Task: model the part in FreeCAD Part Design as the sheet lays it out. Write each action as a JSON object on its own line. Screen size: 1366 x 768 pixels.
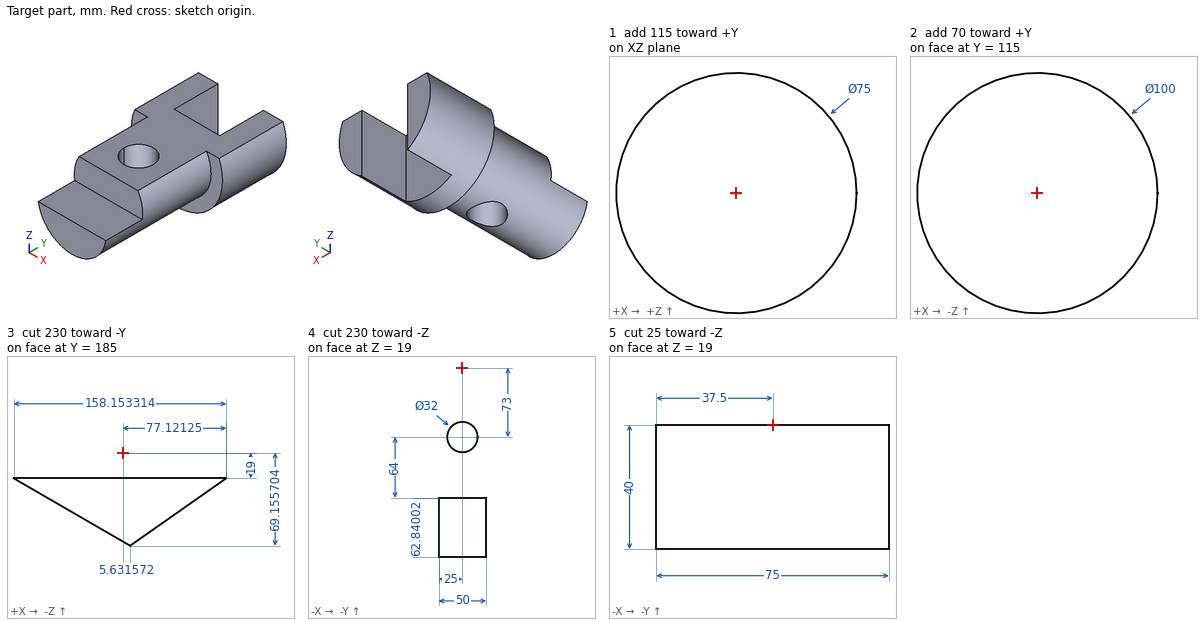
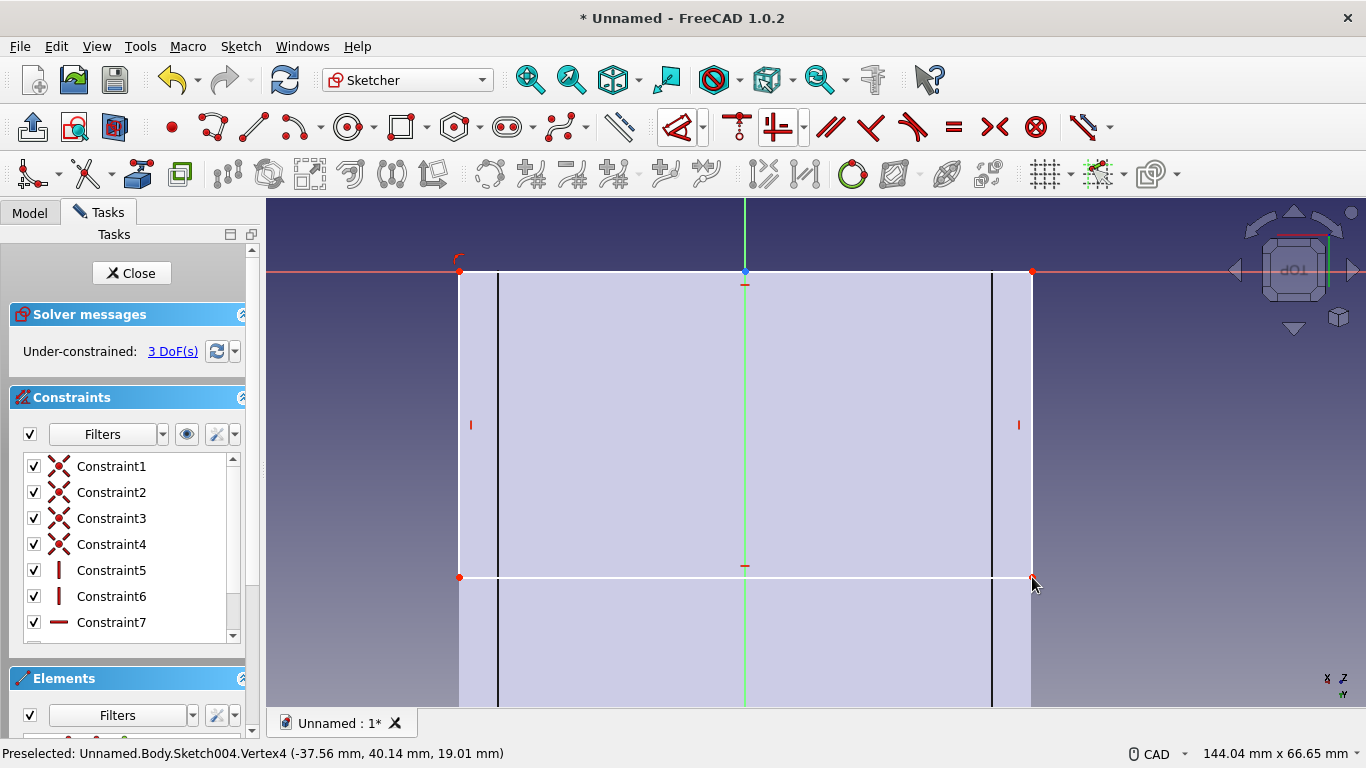
{"action": "left_click", "coordinate": [459, 363]}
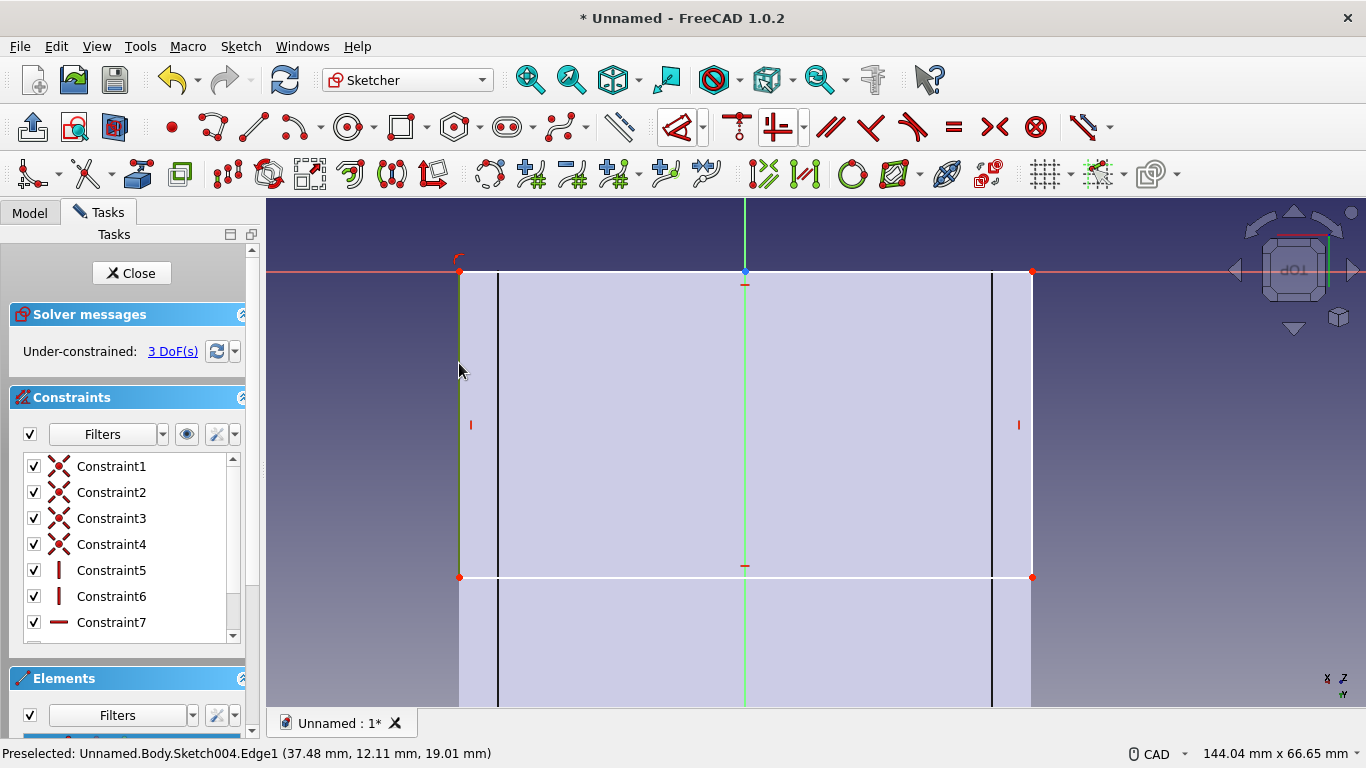
{"action": "left_click", "coordinate": [702, 128]}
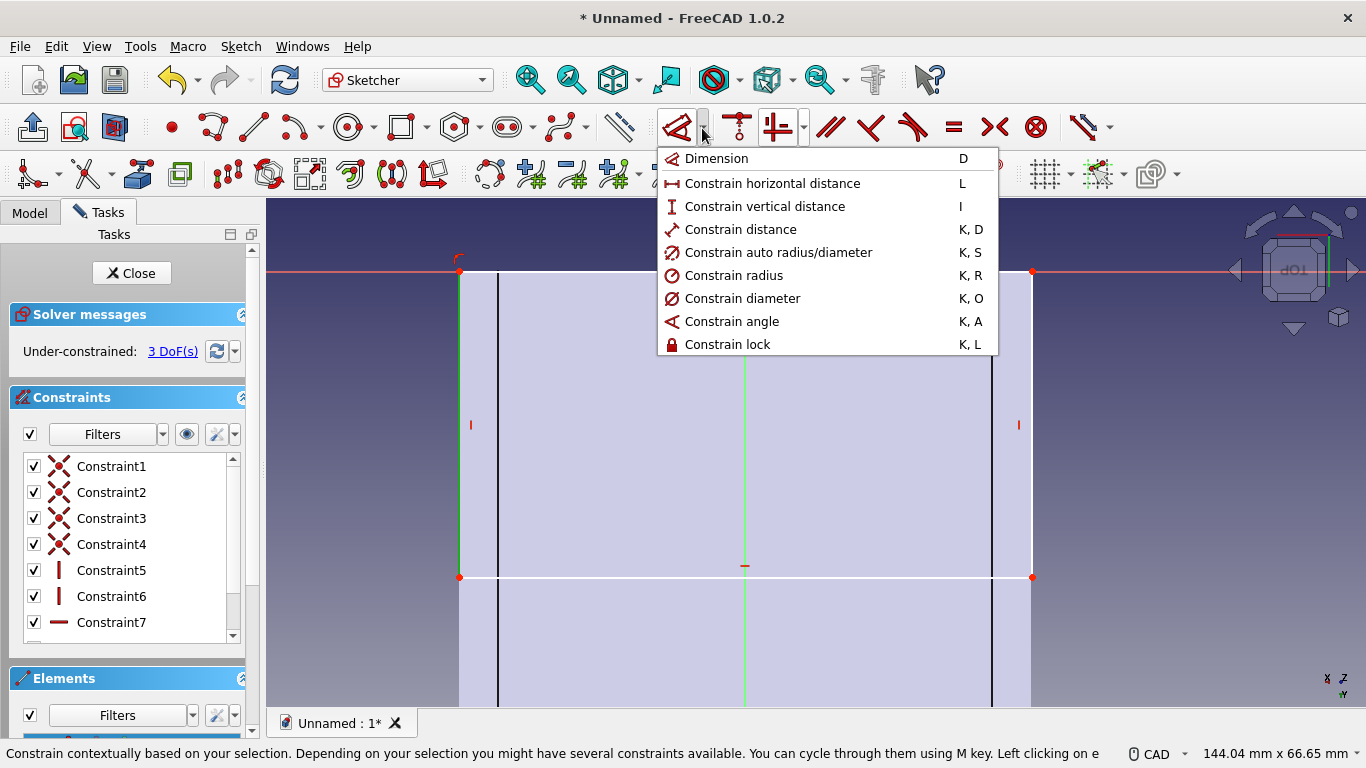
{"action": "left_click", "coordinate": [828, 206]}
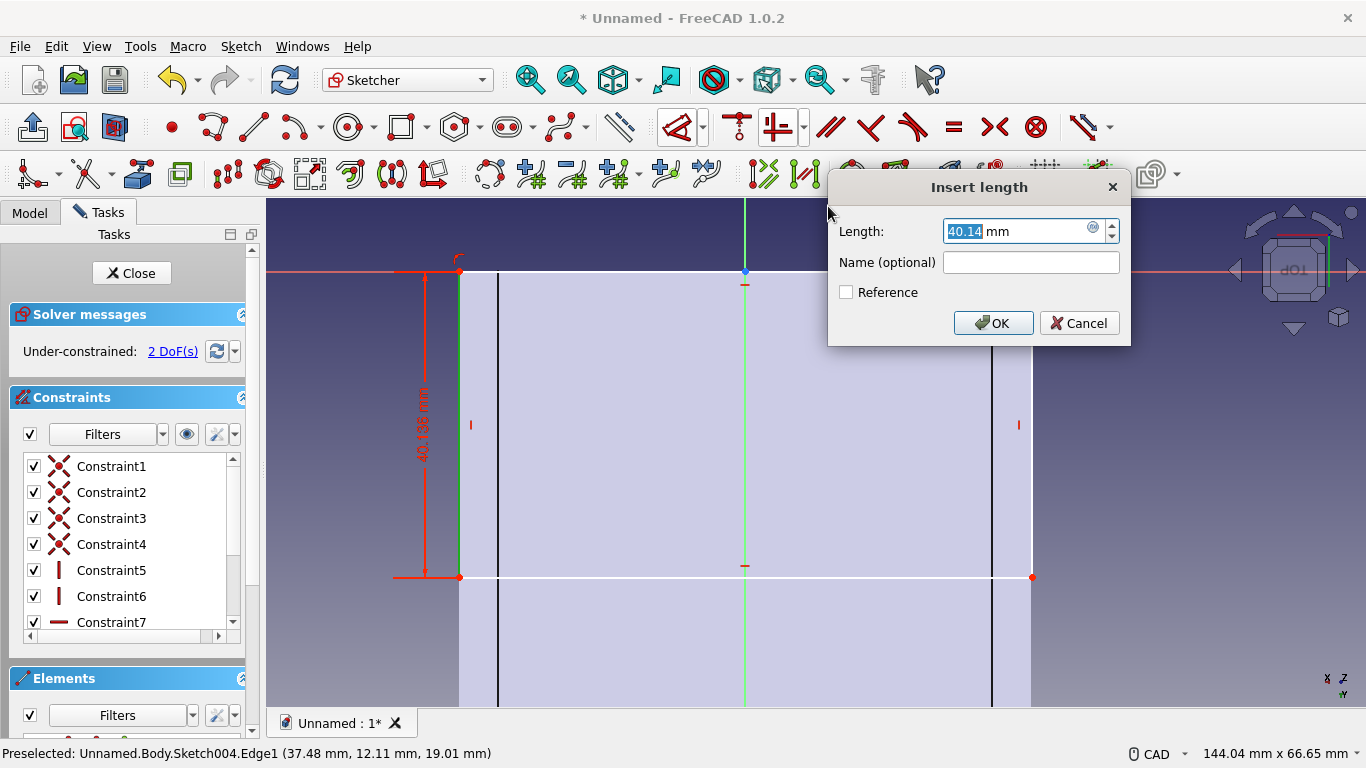
{"action": "type", "text": "40"}
{"action": "key", "text": "Return"}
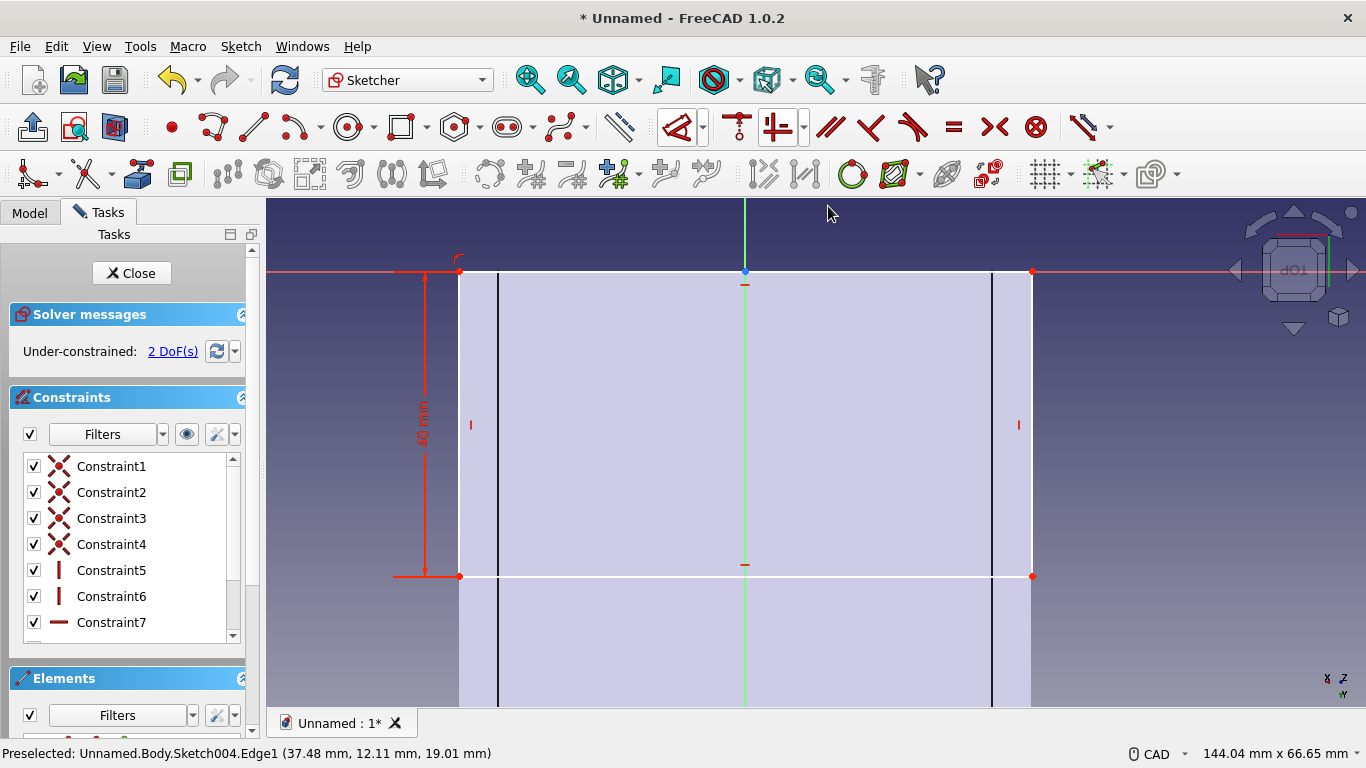
{"action": "left_click", "coordinate": [631, 577]}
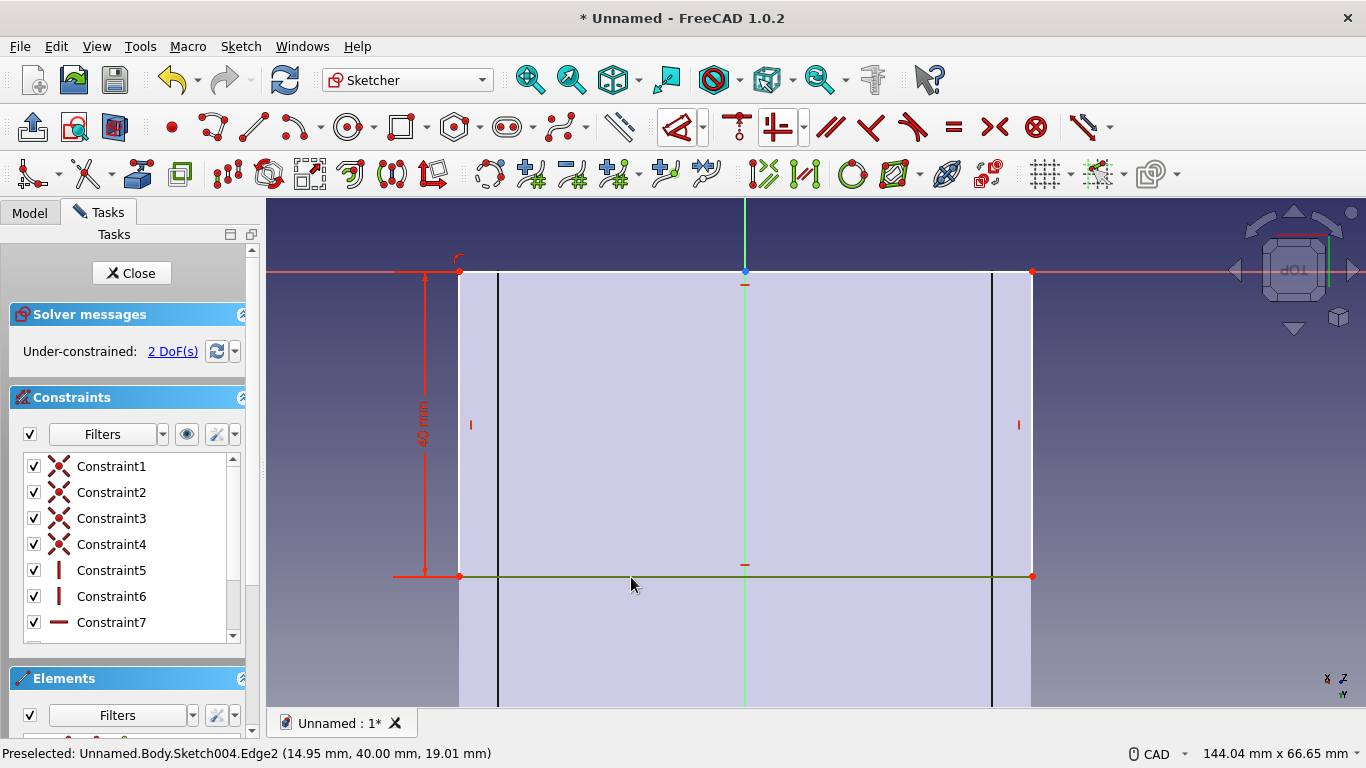
{"action": "left_click", "coordinate": [702, 128]}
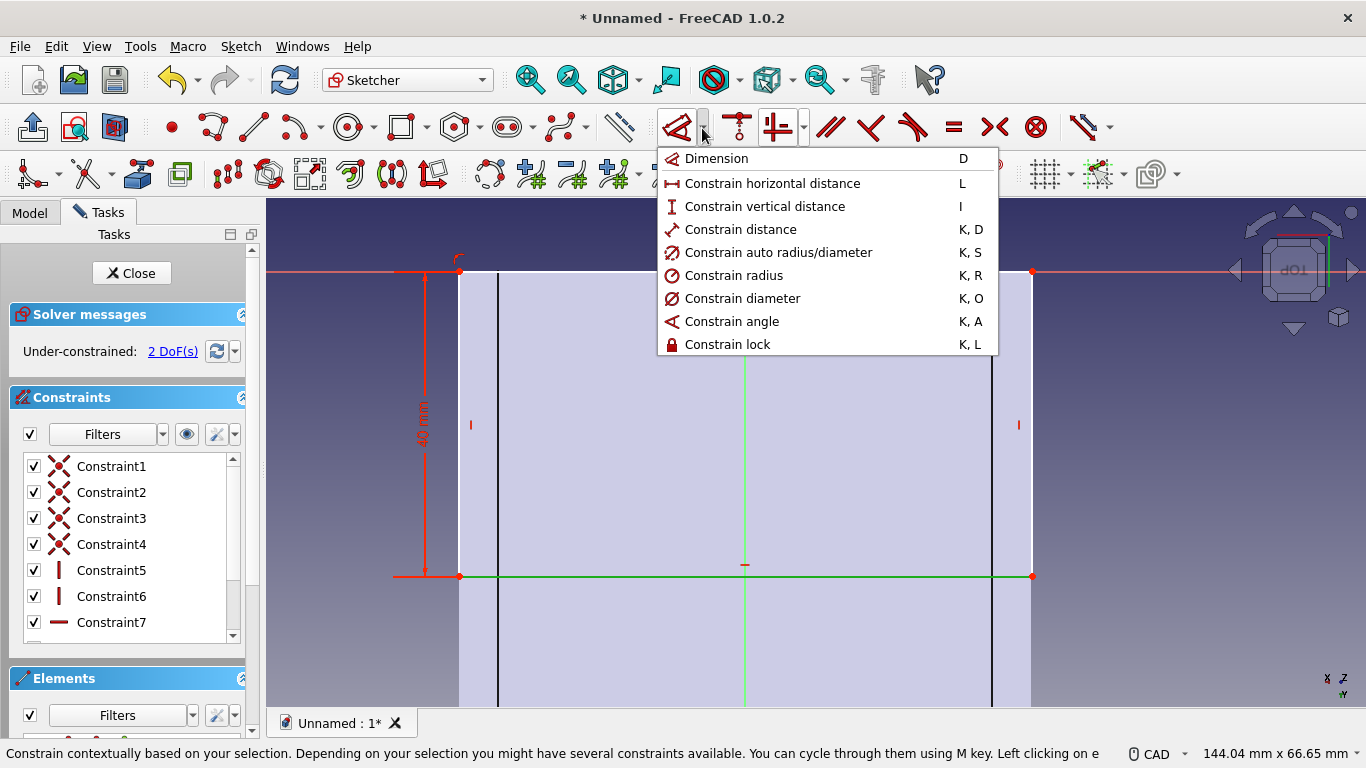
{"action": "left_click", "coordinate": [828, 184]}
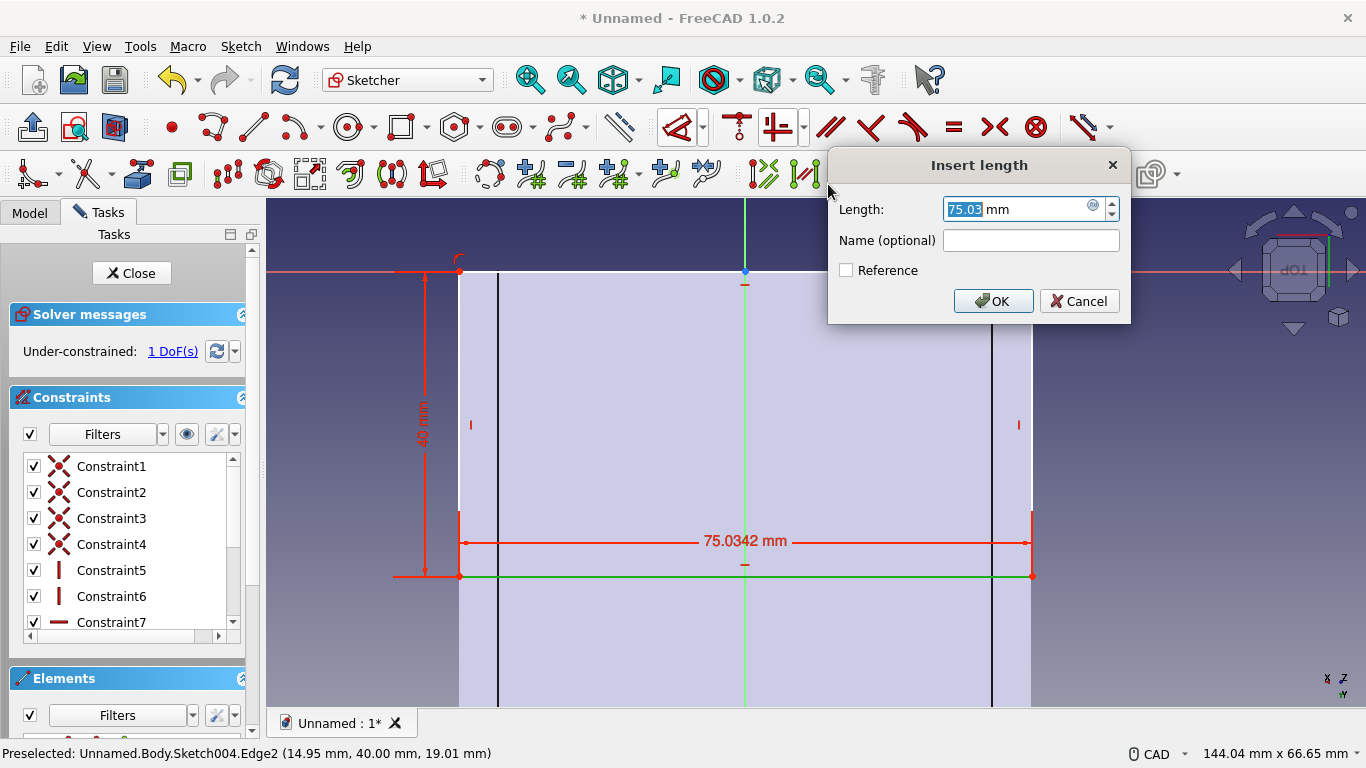
{"action": "type", "text": "75"}
{"action": "key", "text": "Return"}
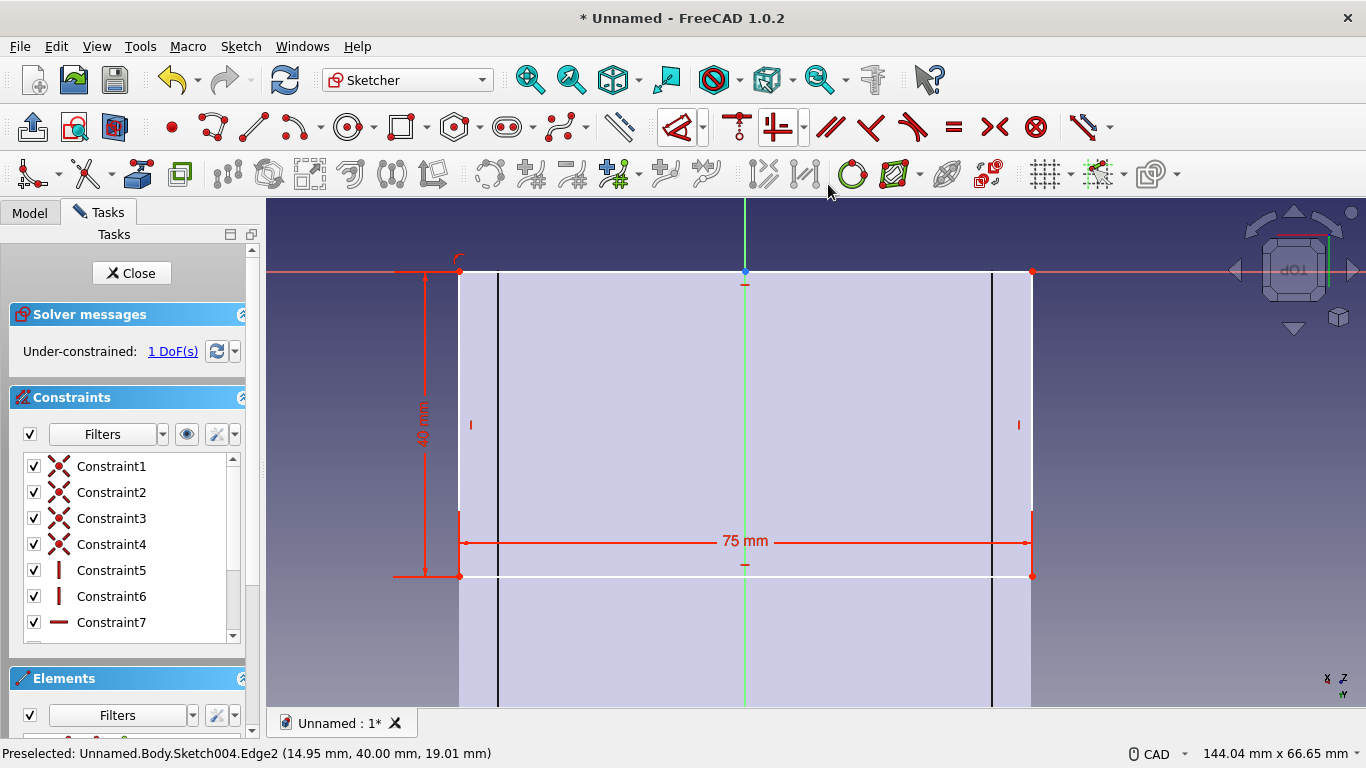
{"action": "left_click", "coordinate": [459, 272]}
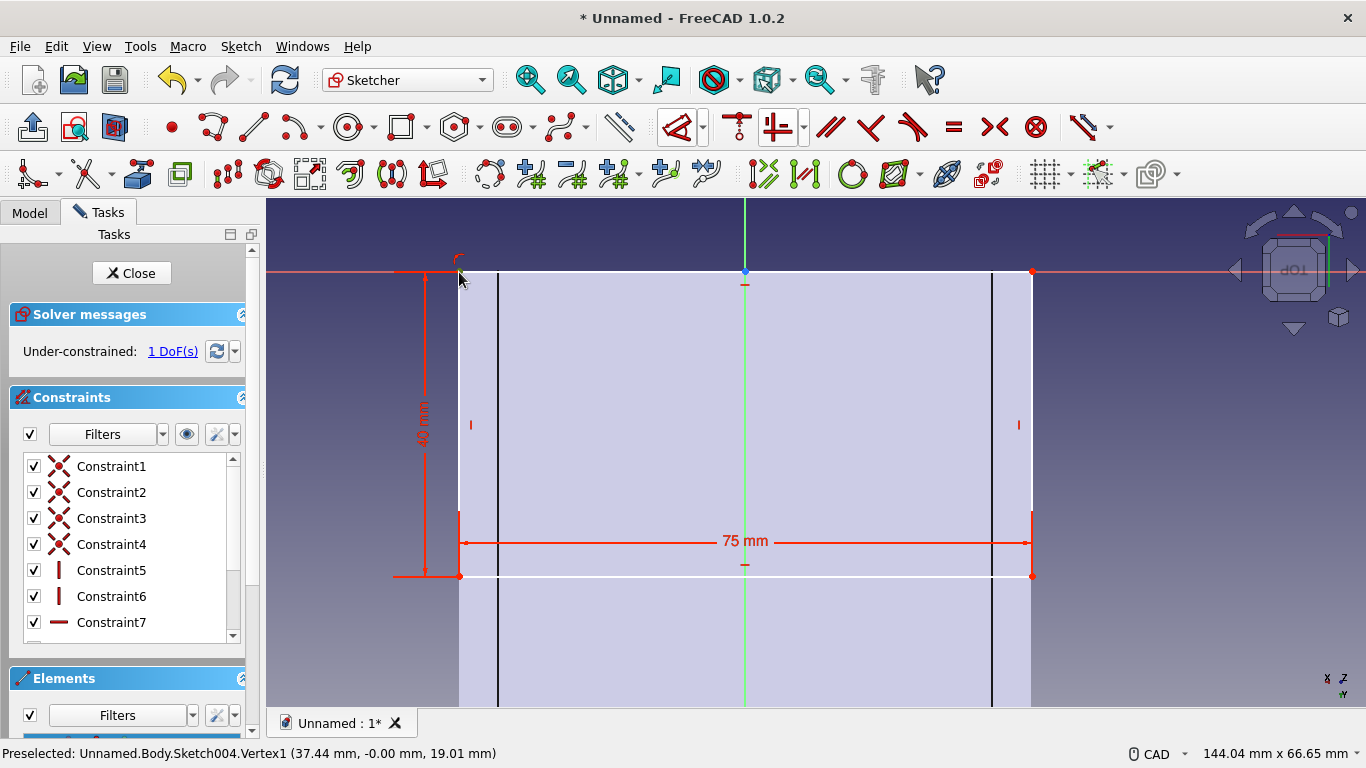
{"action": "left_click", "coordinate": [702, 128]}